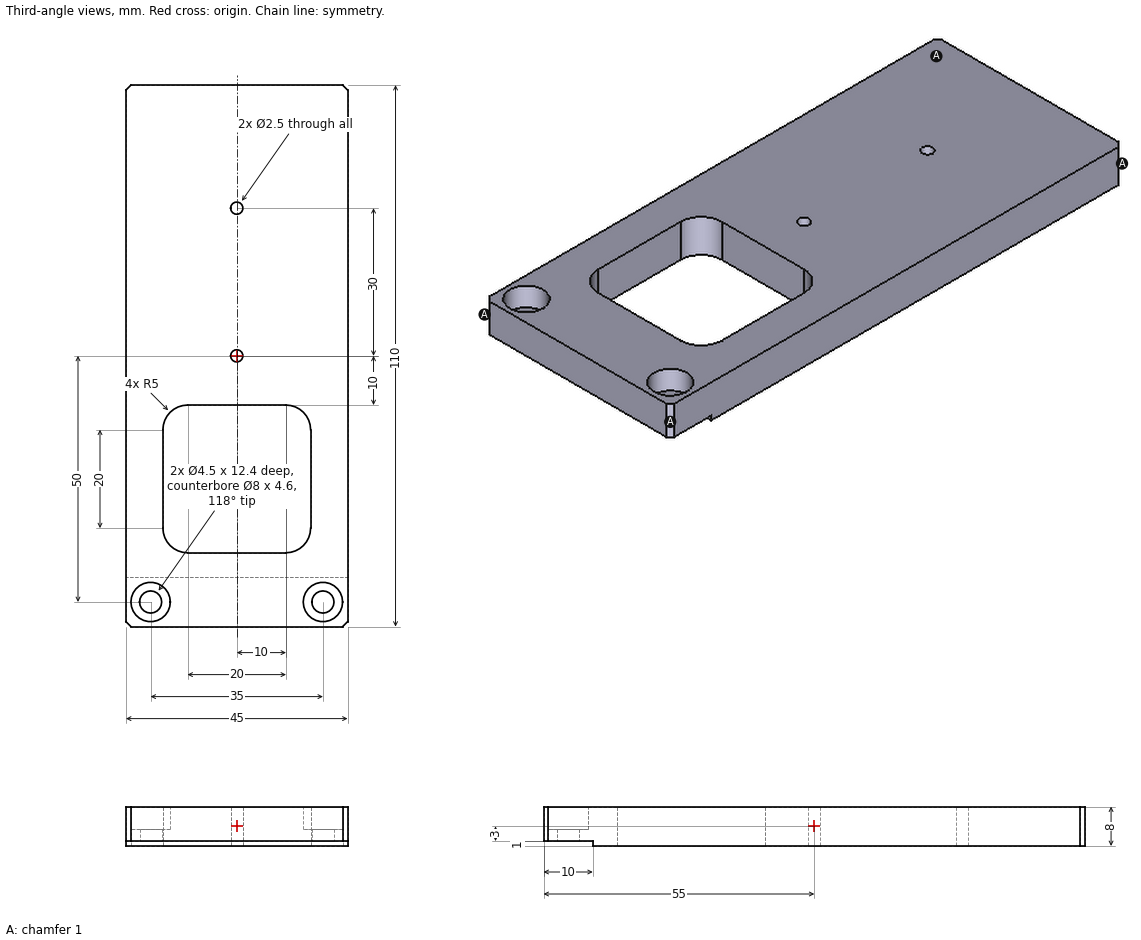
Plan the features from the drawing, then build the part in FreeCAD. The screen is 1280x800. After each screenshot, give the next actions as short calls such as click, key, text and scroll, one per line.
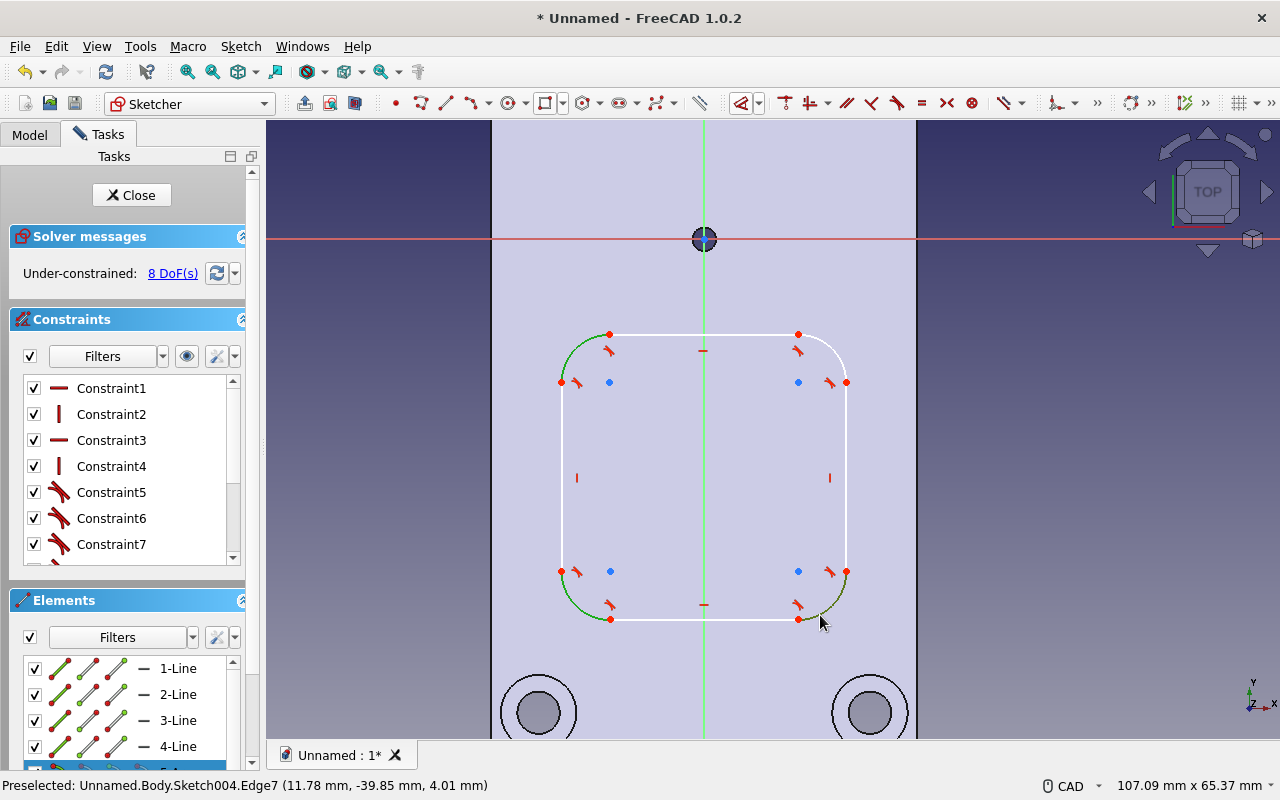
click(841, 361)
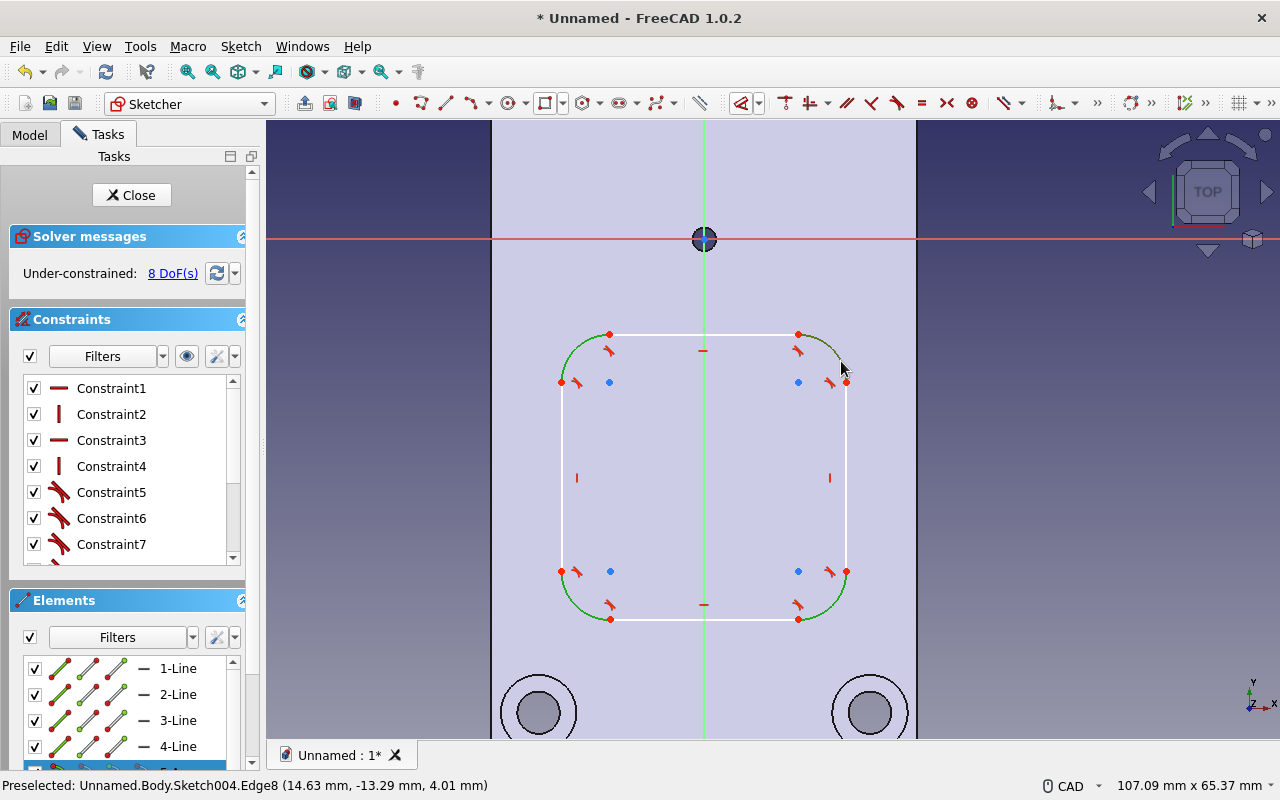
click(922, 104)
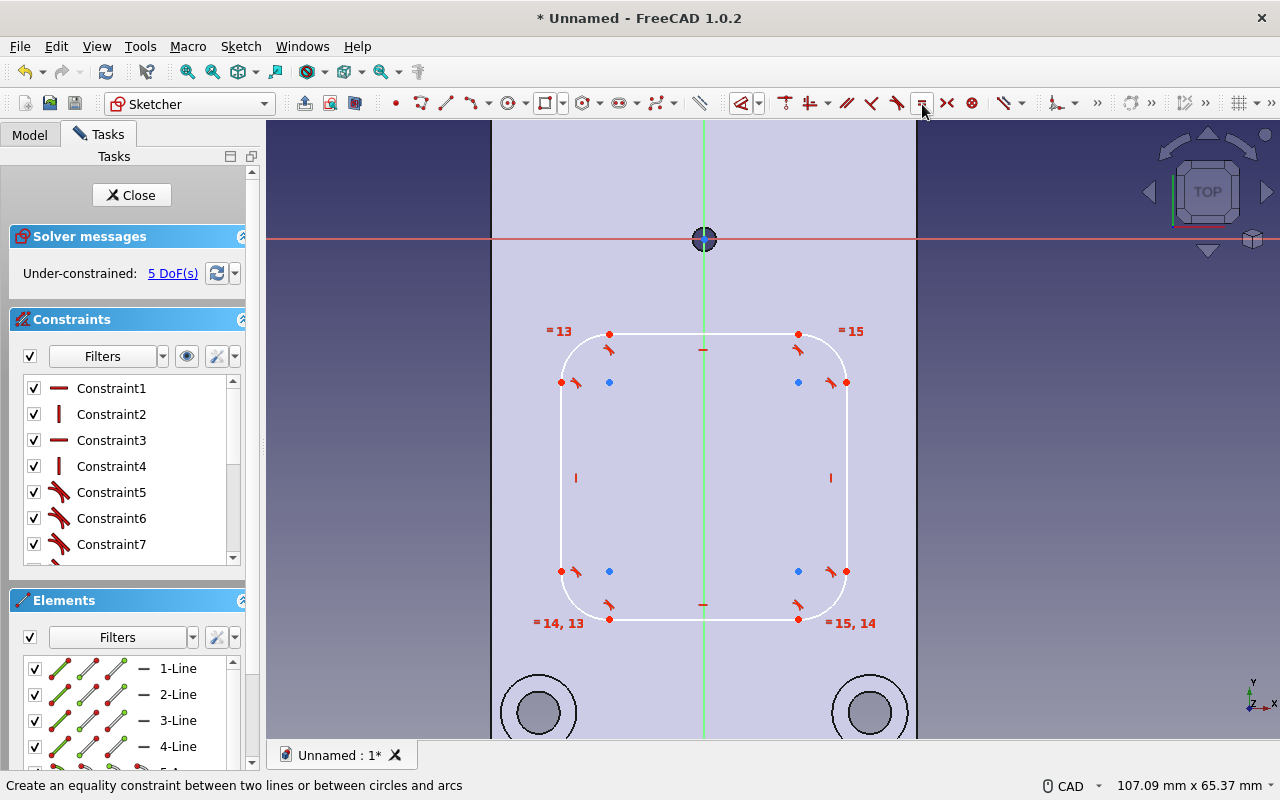
click(588, 340)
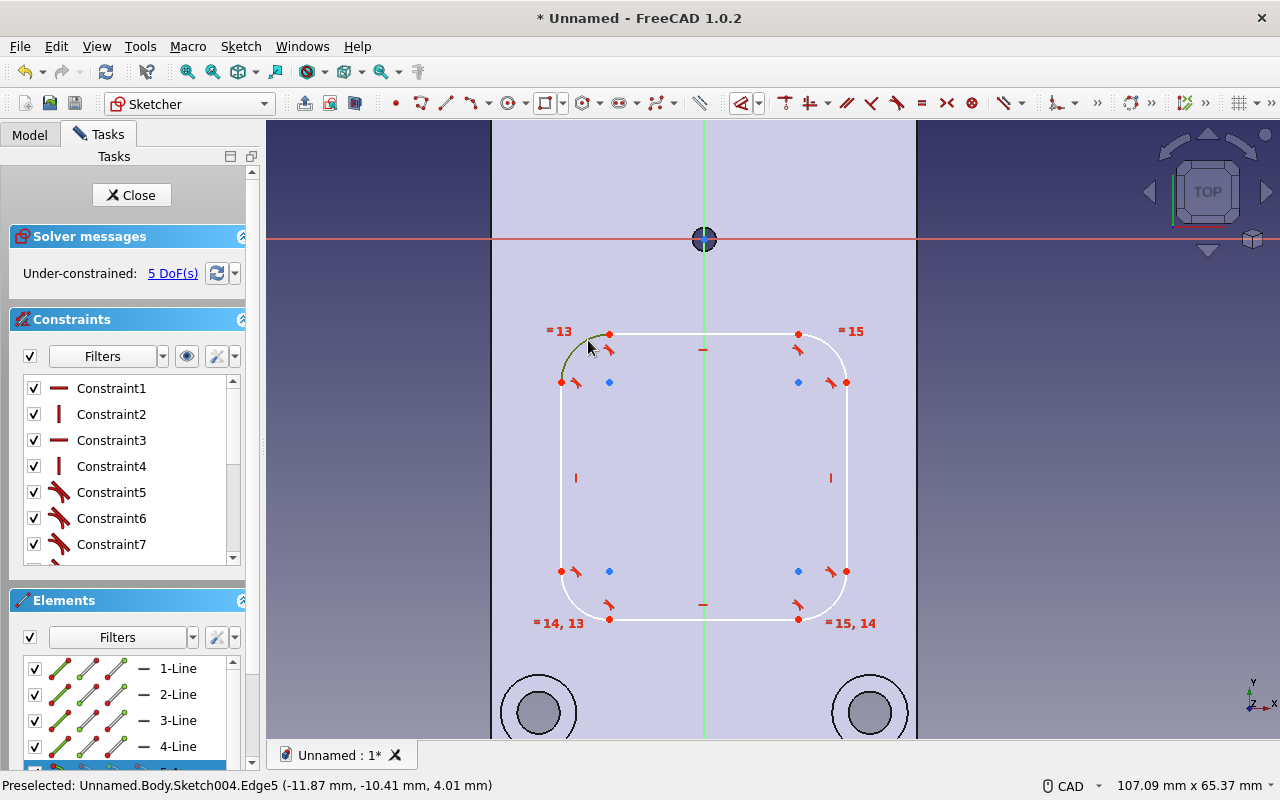
click(758, 104)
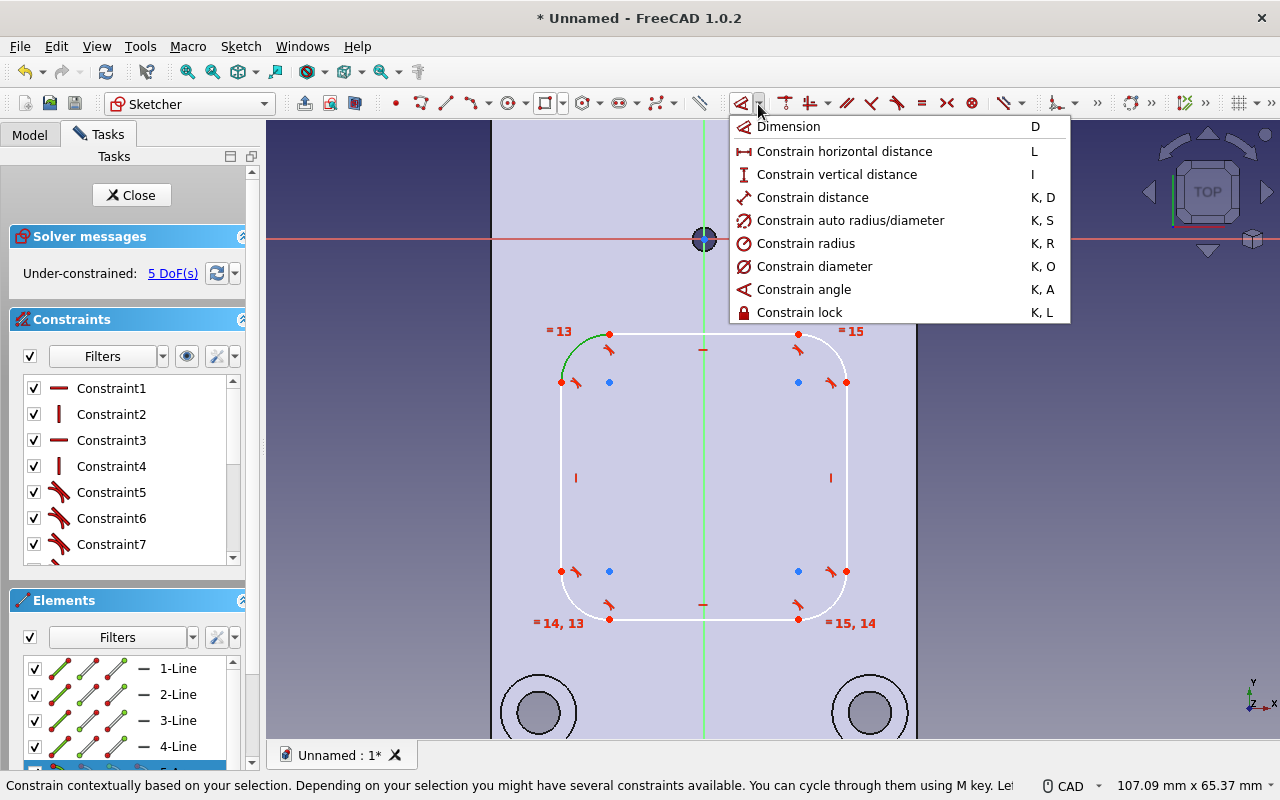
click(900, 244)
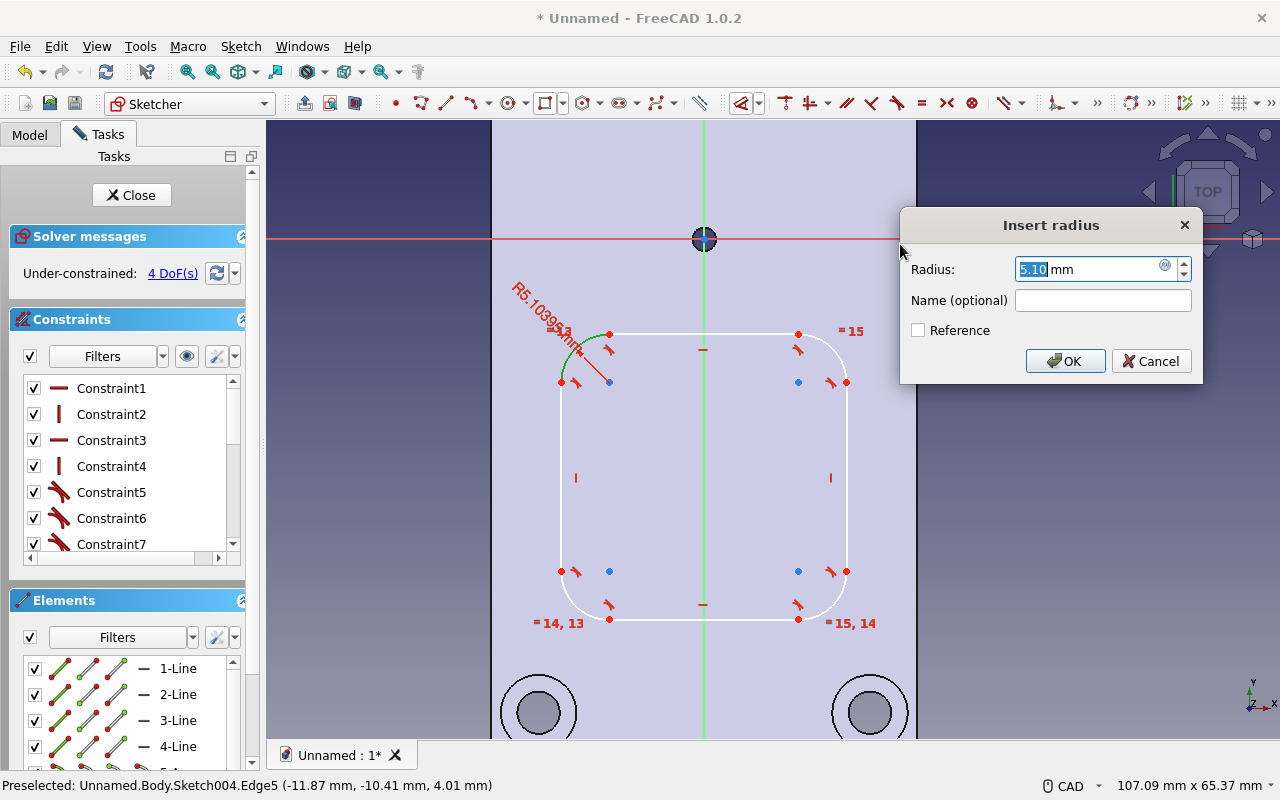
text(5)
key(Return)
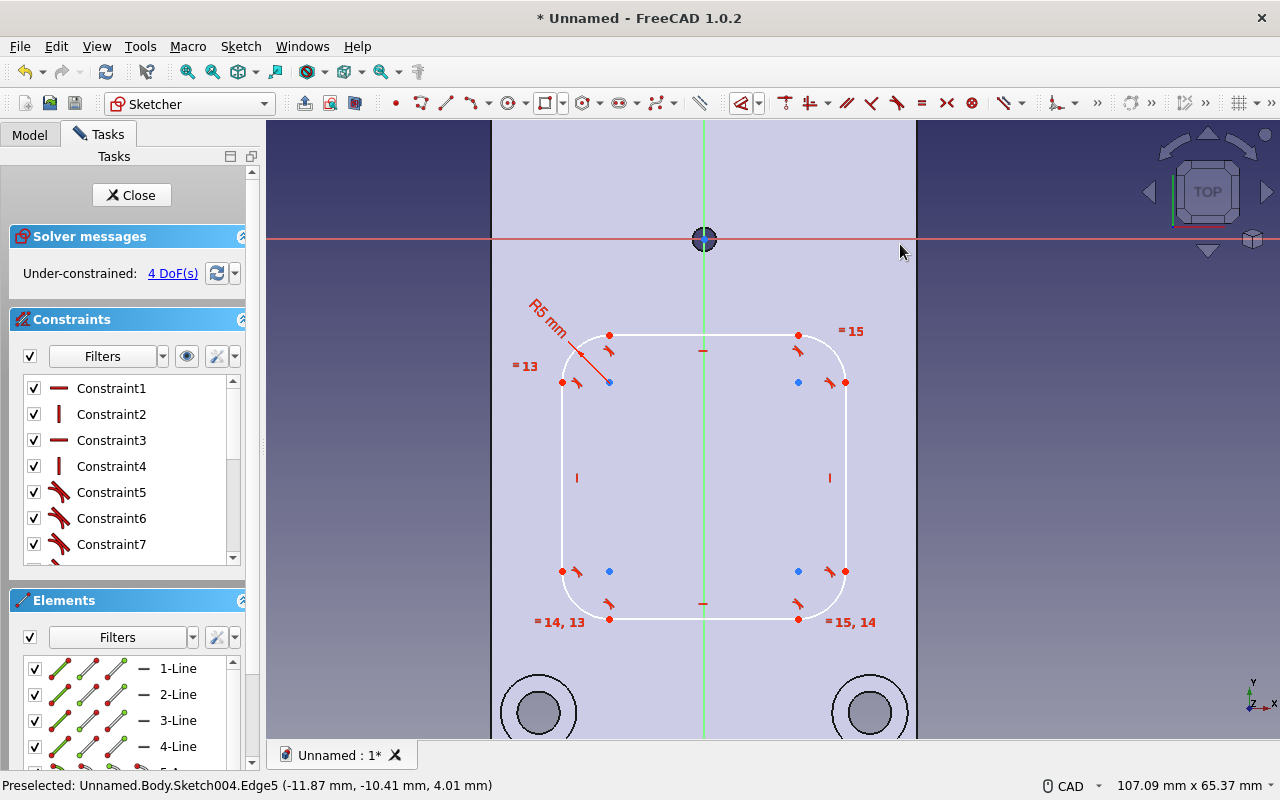
click(742, 335)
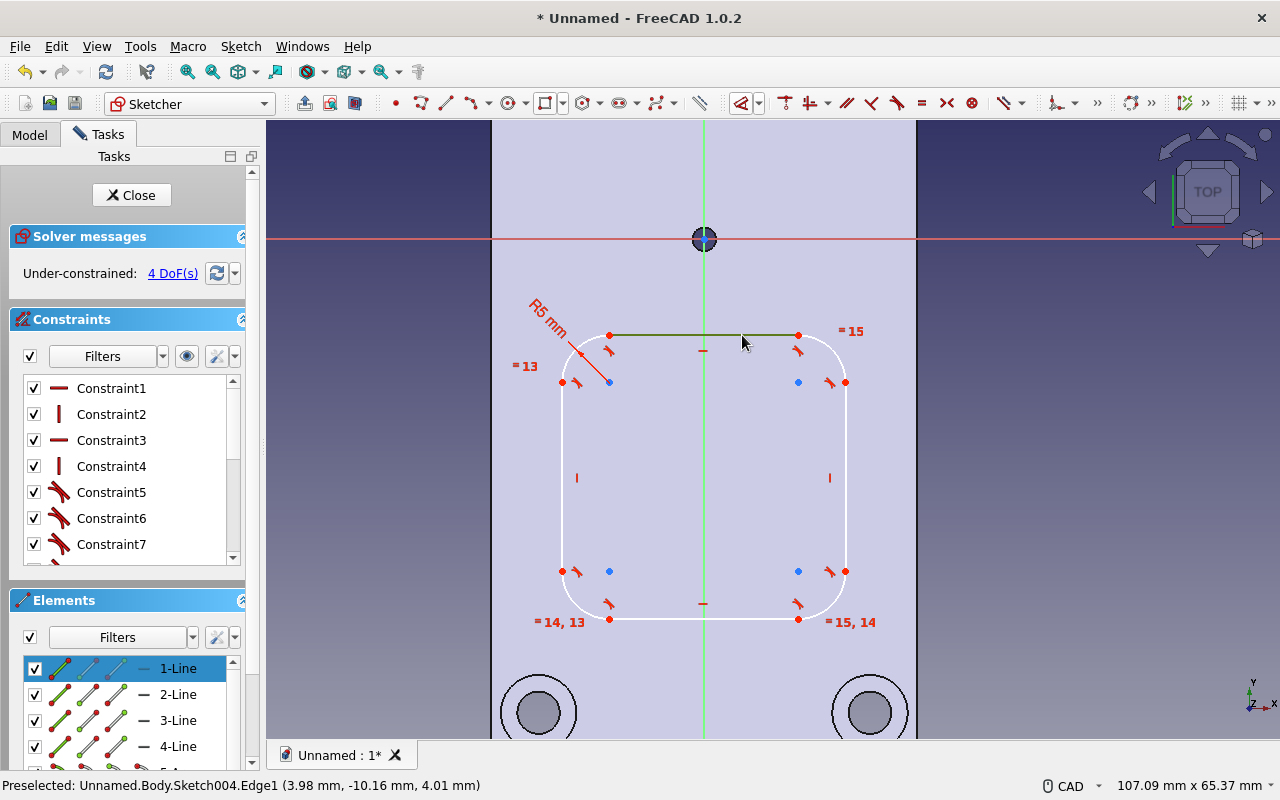
click(758, 104)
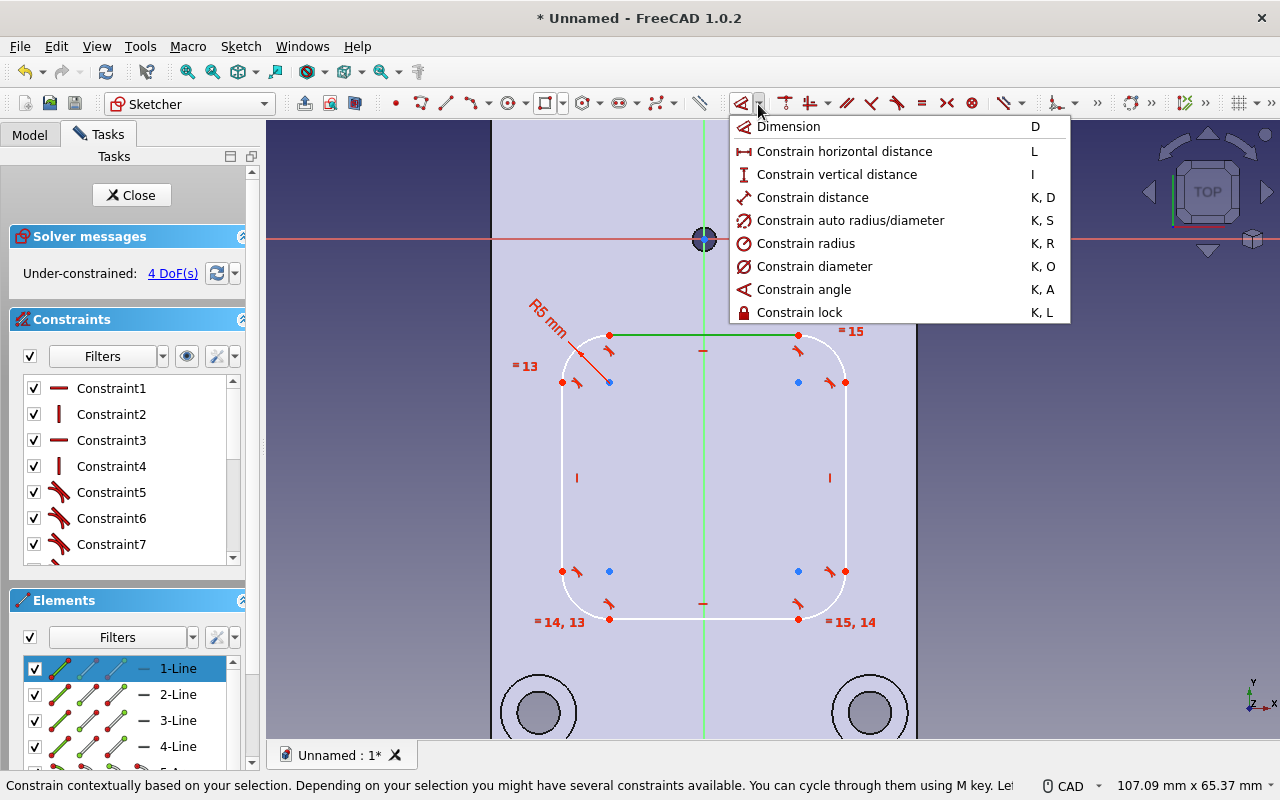
click(900, 152)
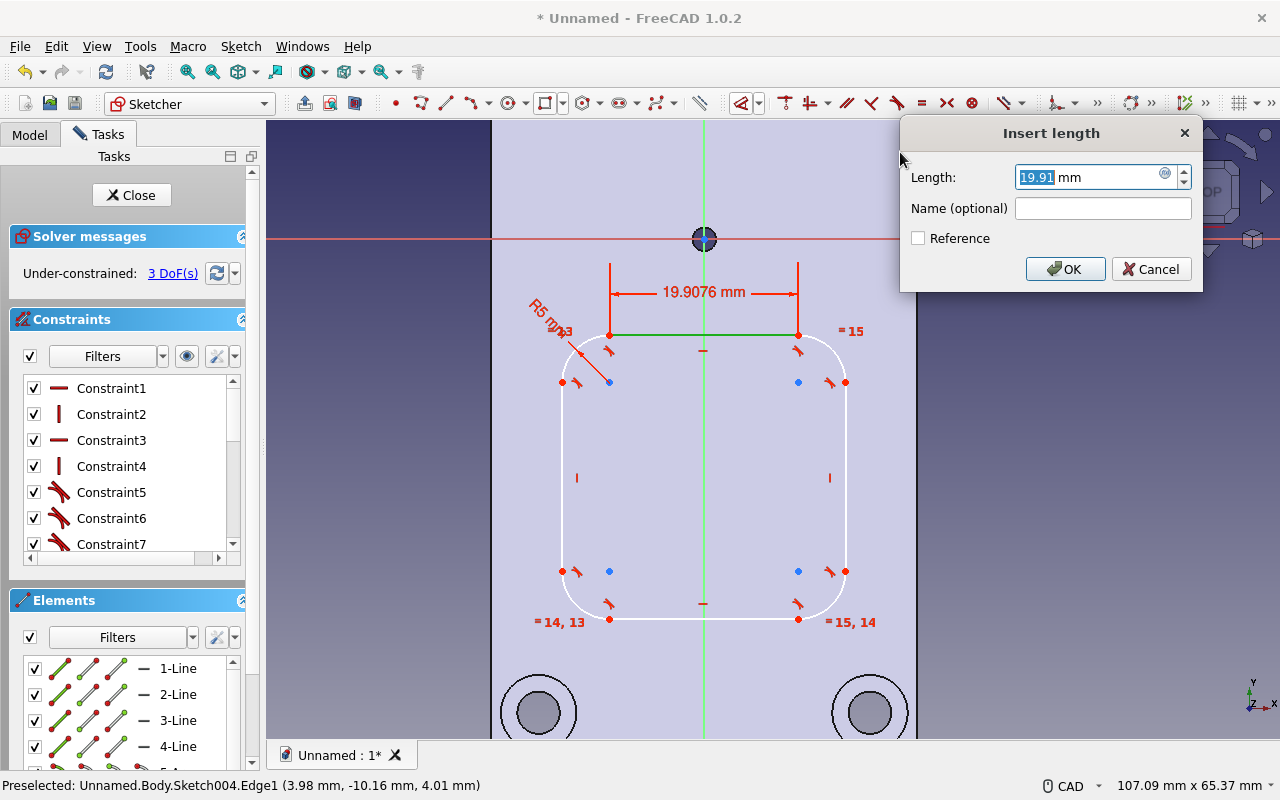
text(20)
key(Return)